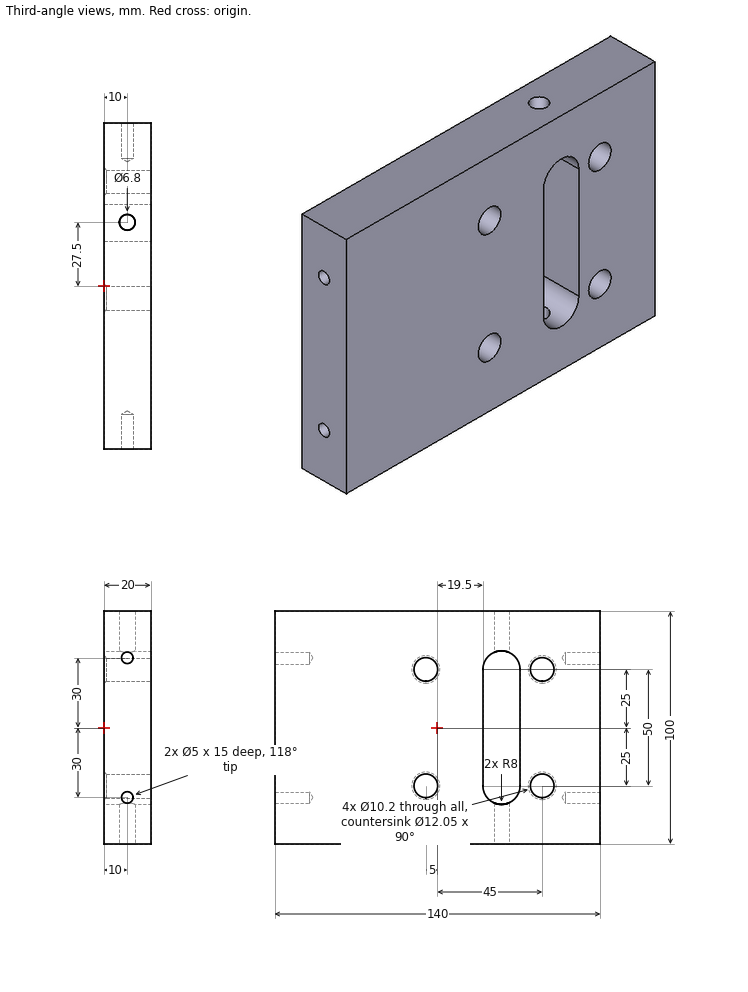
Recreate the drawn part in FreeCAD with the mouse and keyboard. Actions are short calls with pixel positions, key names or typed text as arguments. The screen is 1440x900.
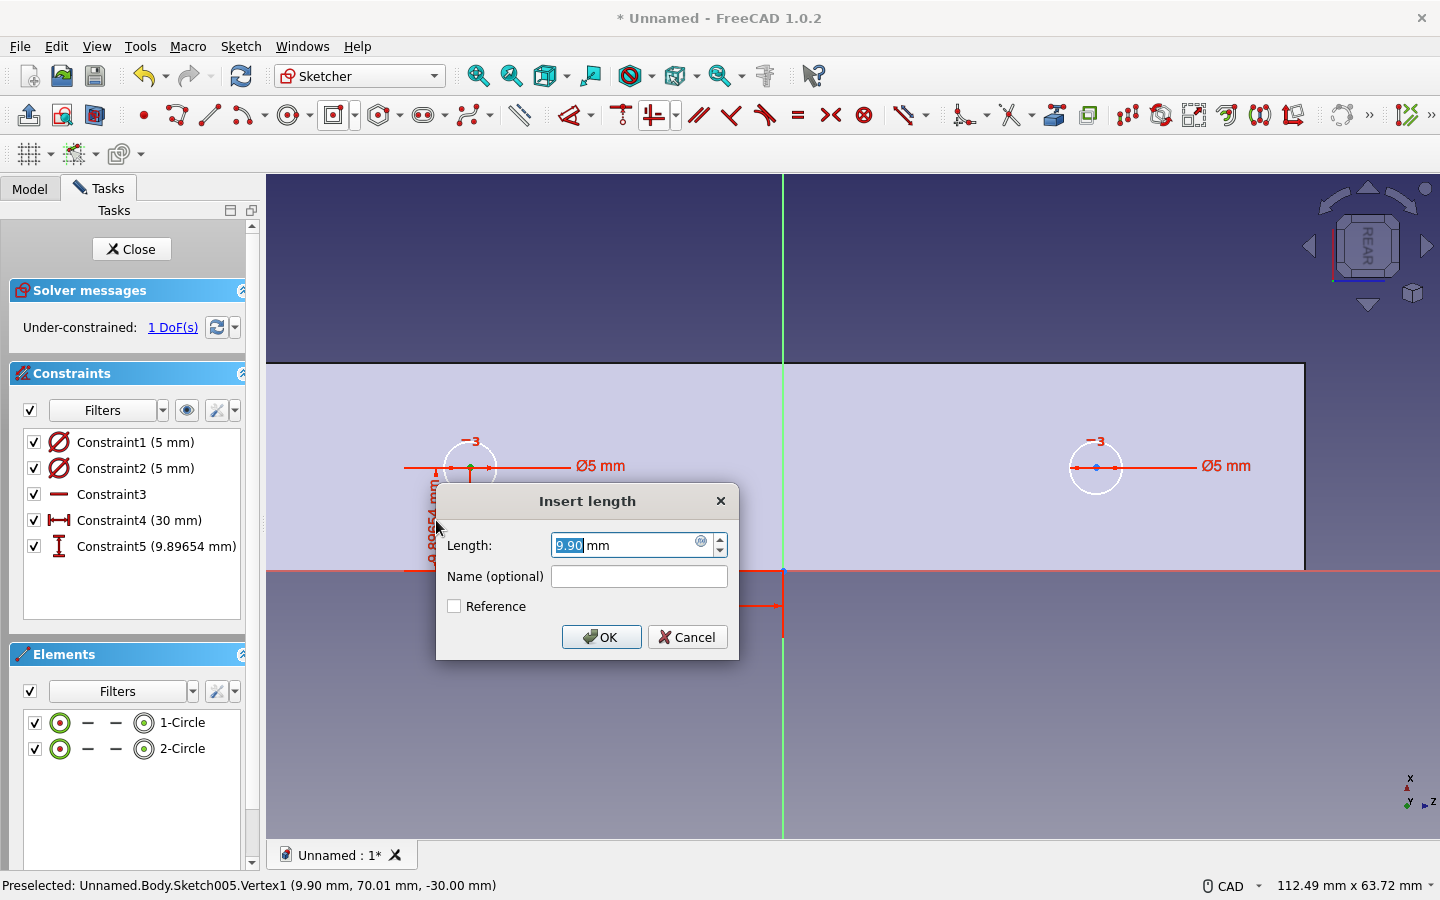
text(10)
key(Return)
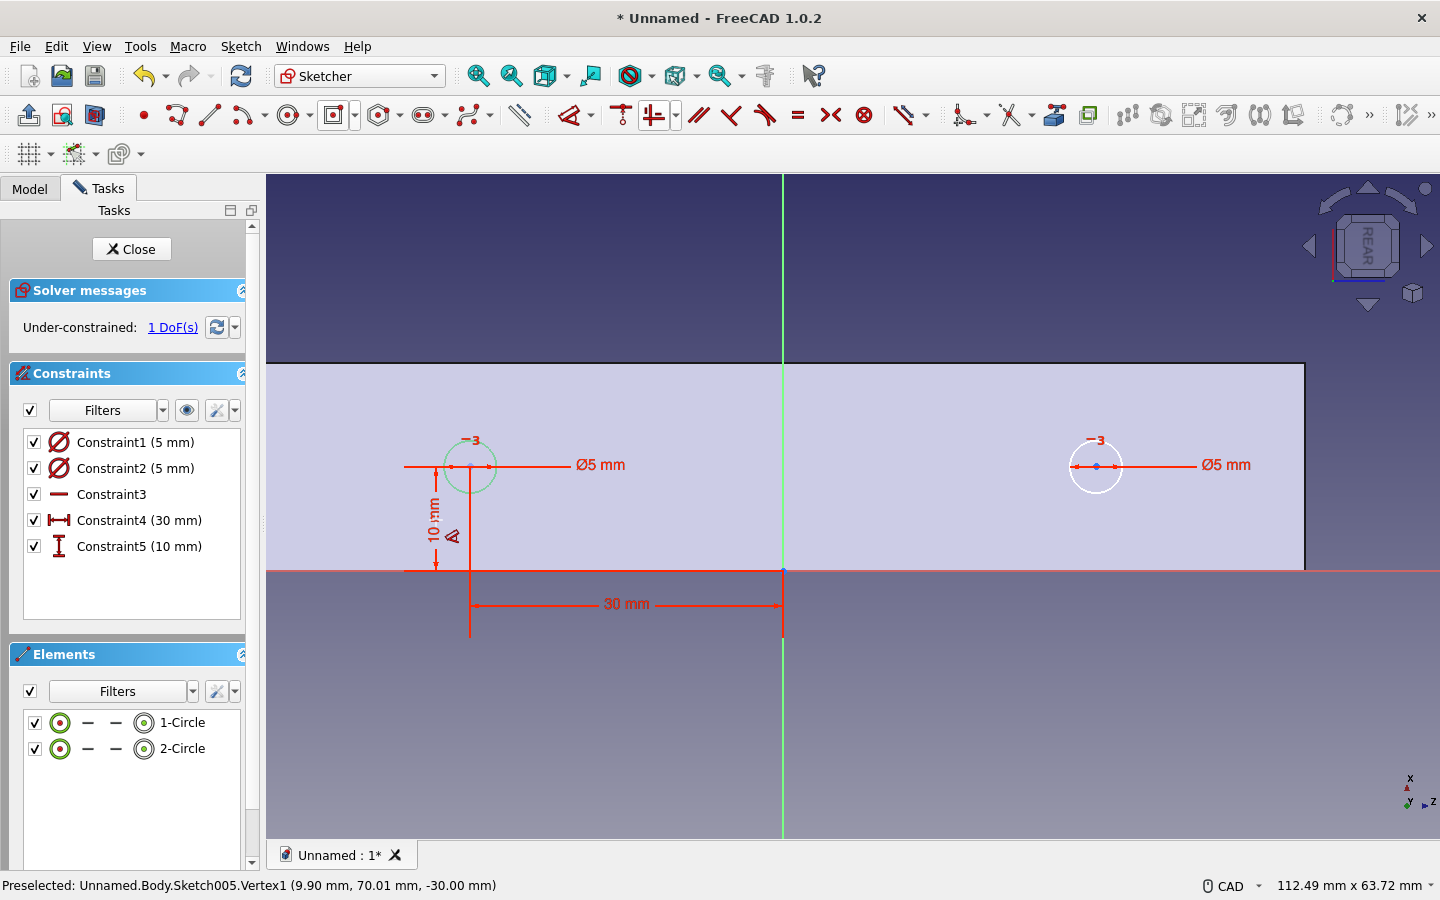
click(1096, 467)
click(940, 605)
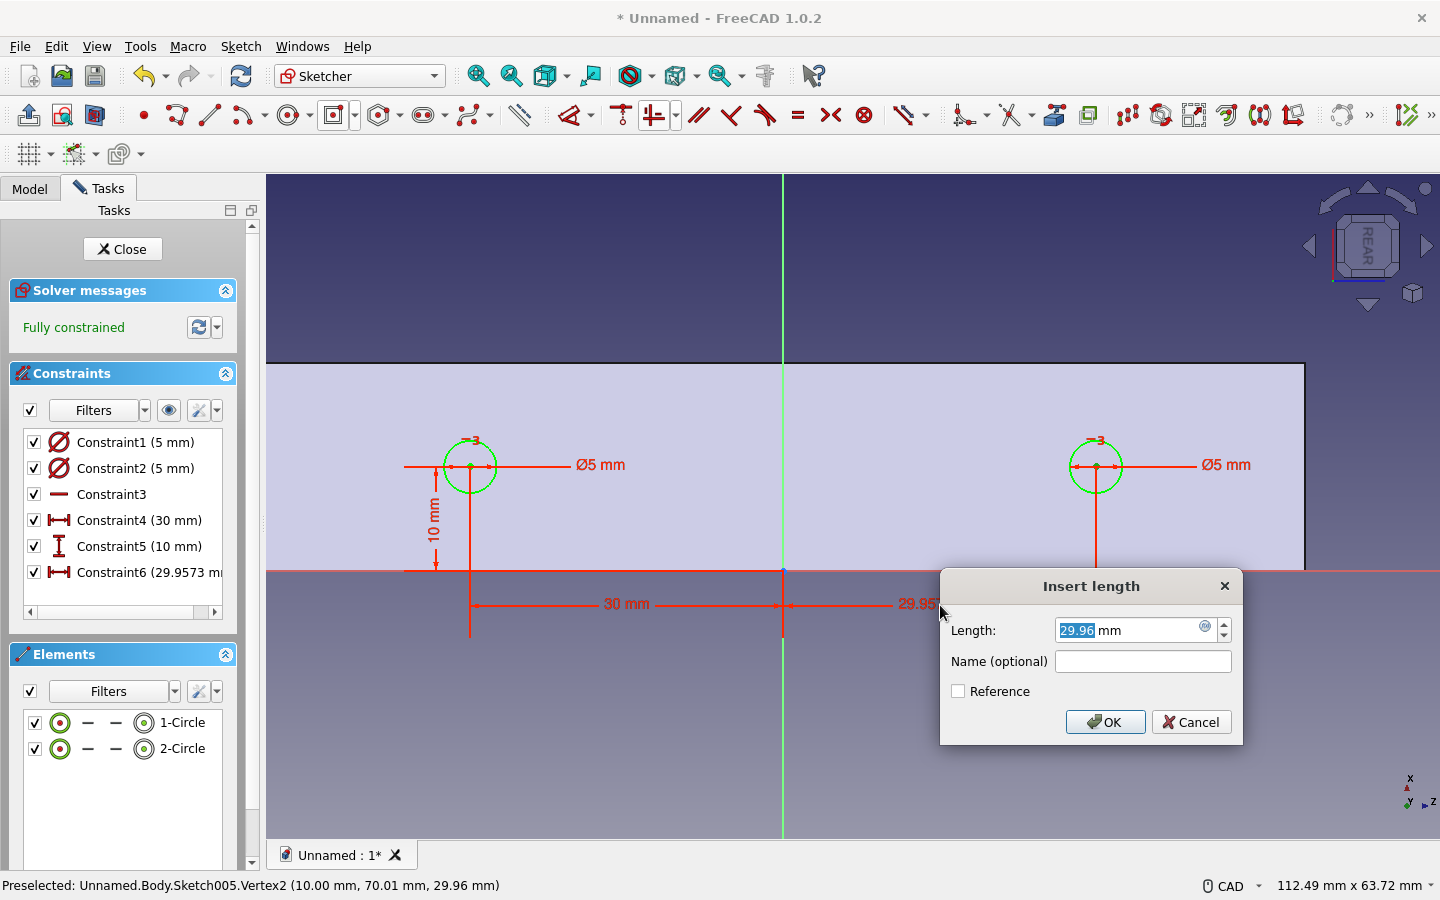
text(30)
key(Return)
key(Escape)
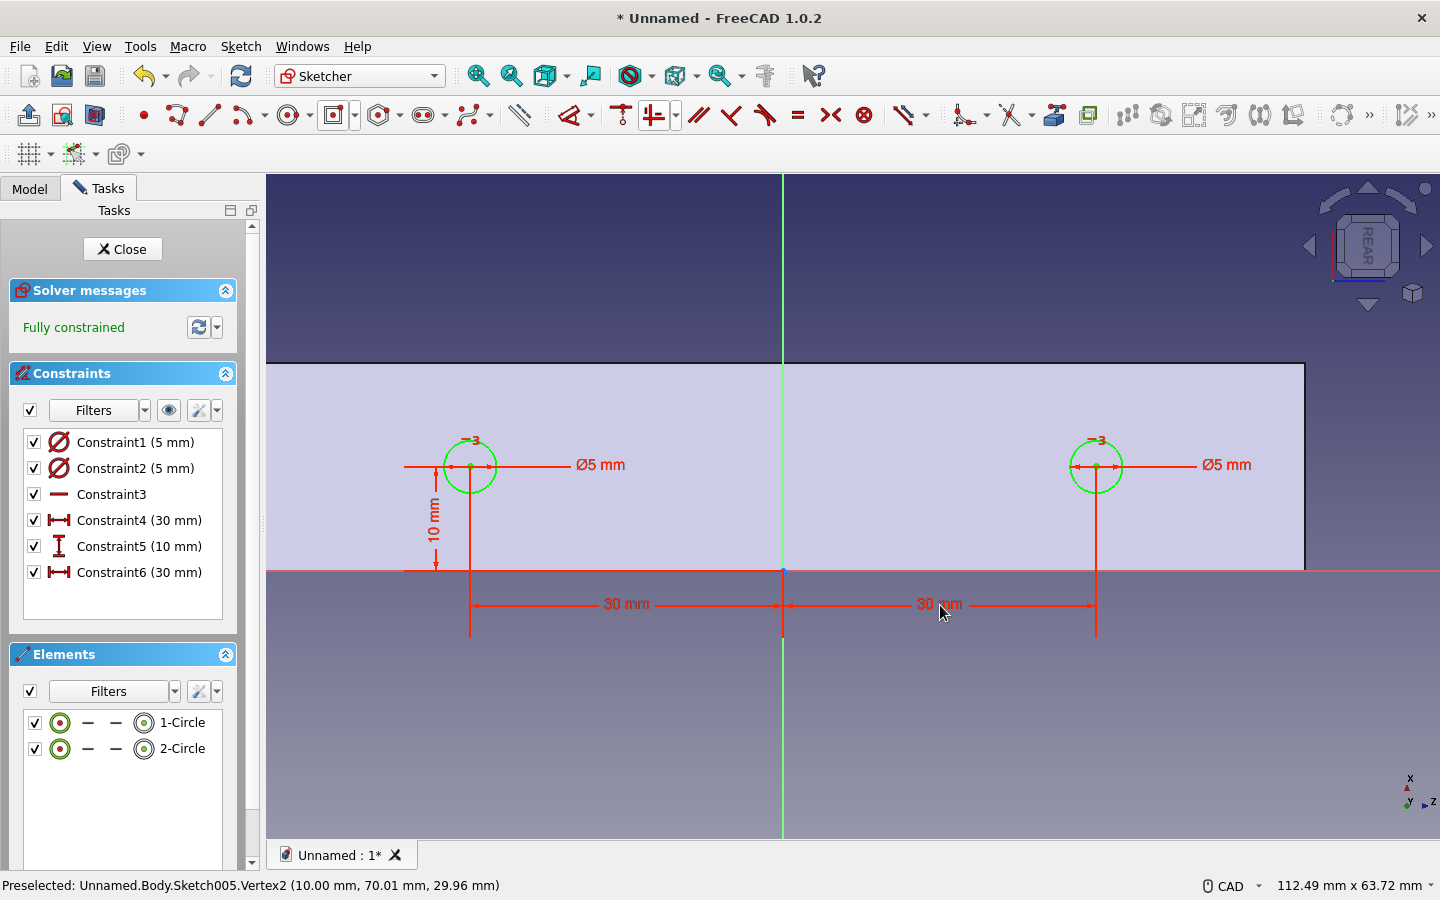
click(123, 249)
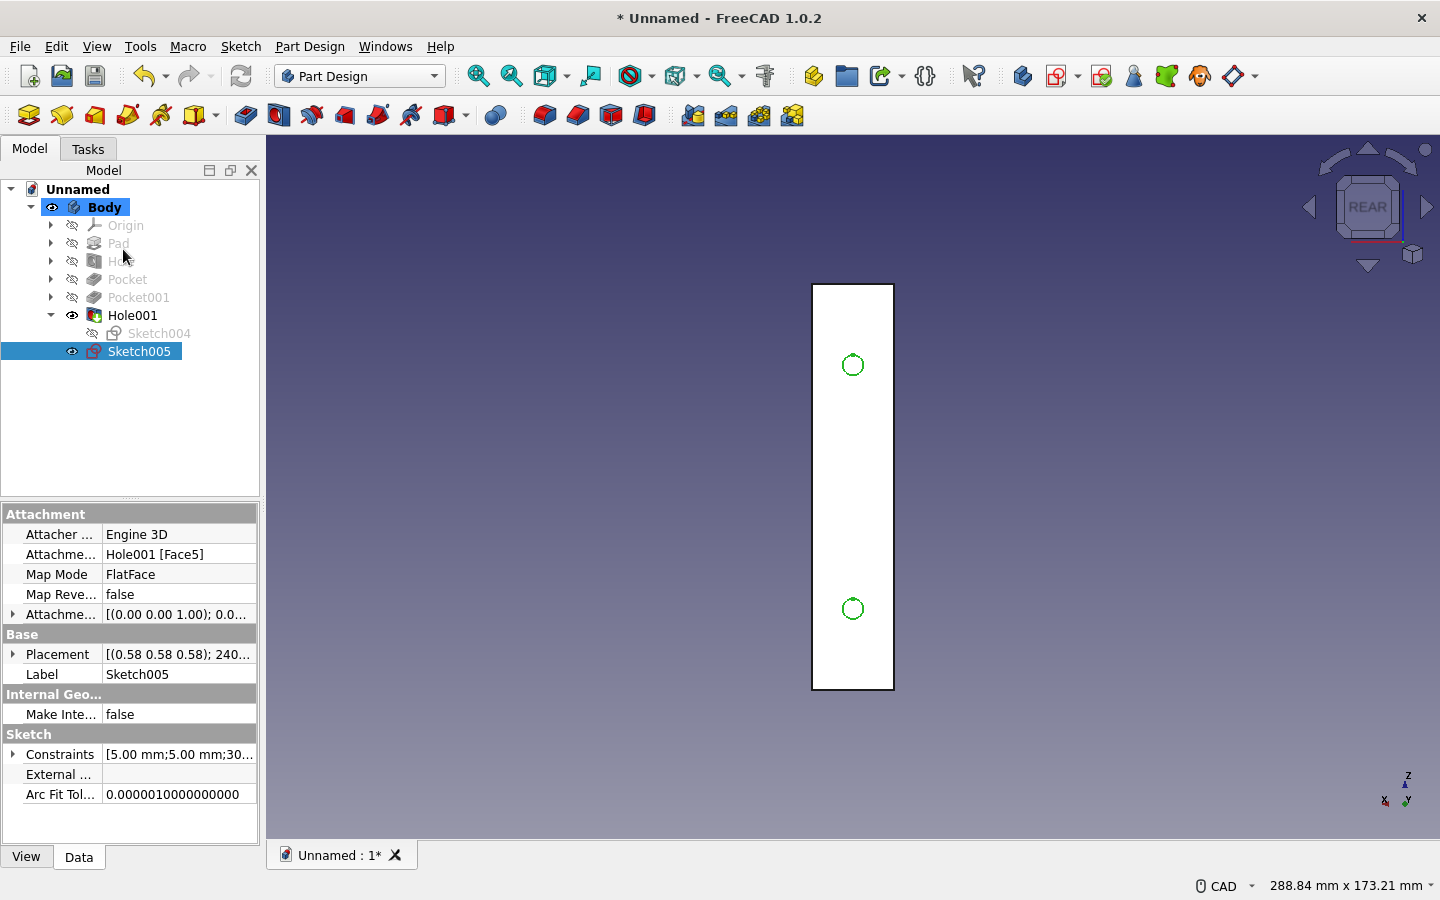
click(279, 116)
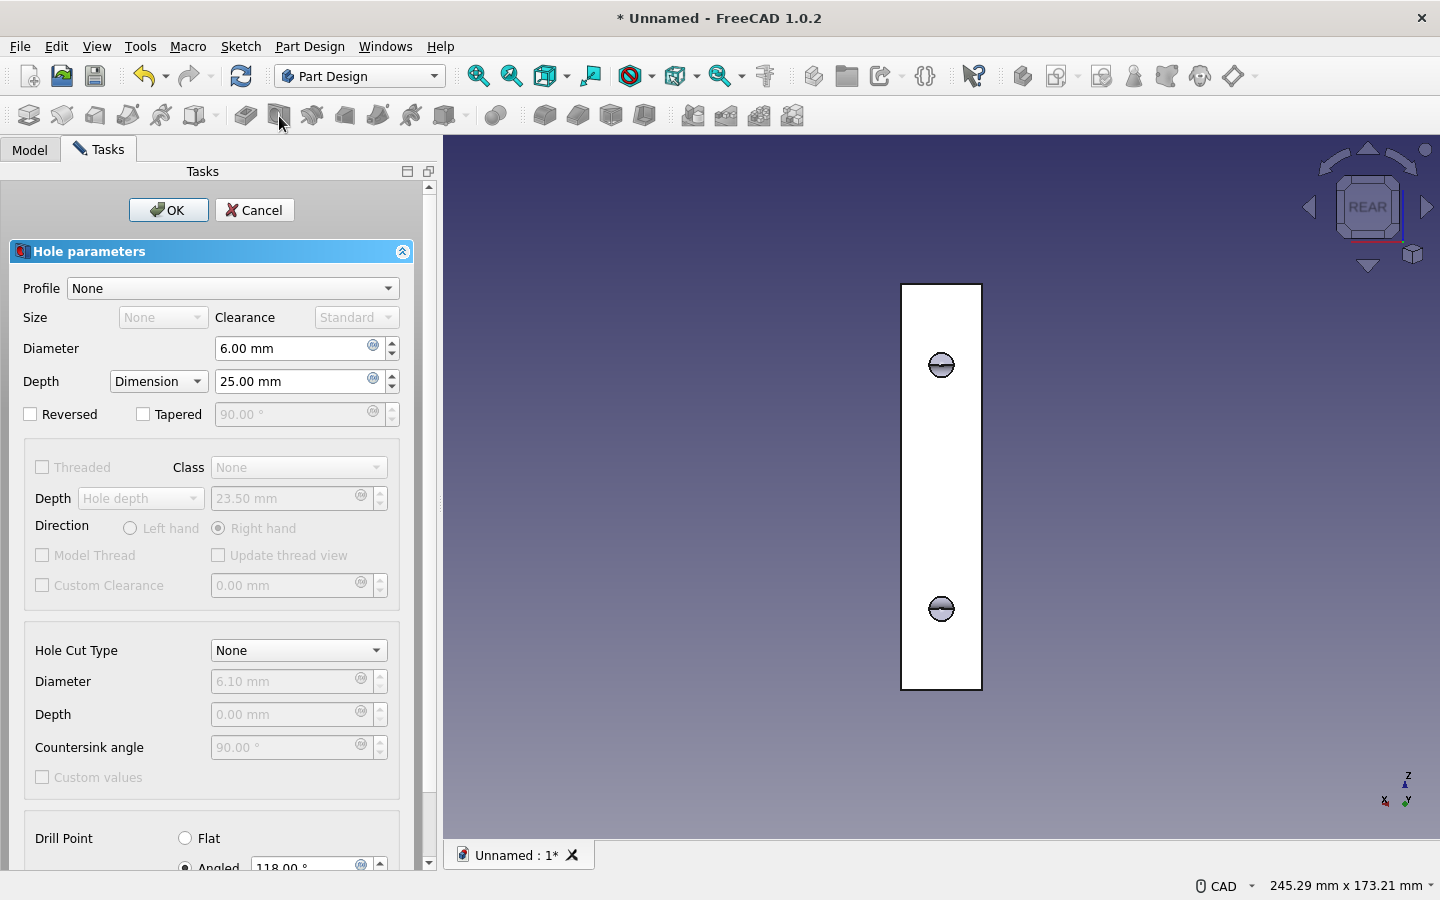
triple_click(300, 348)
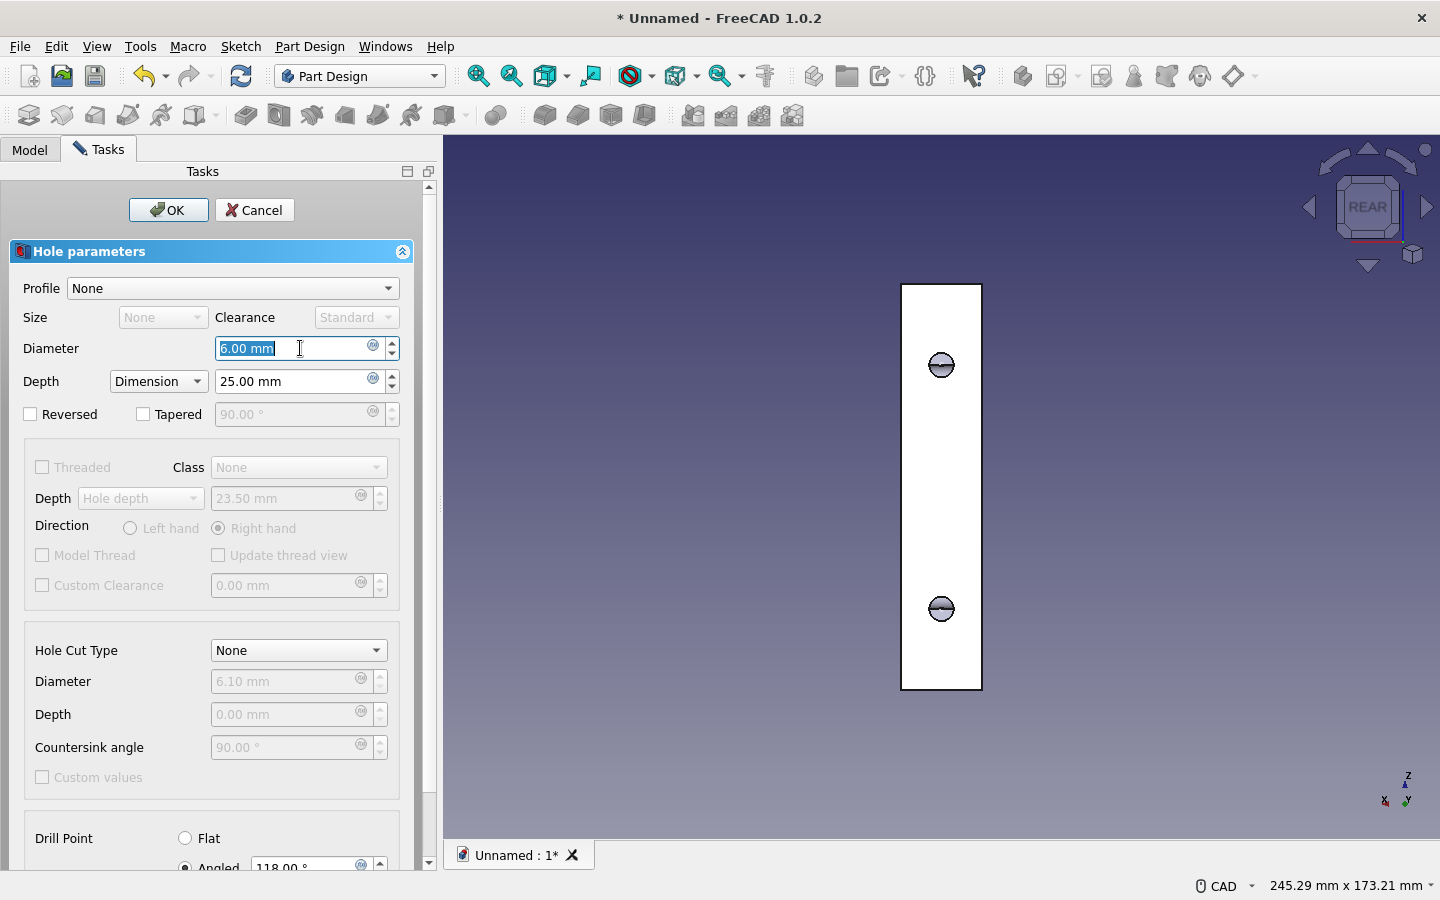
text(5)
key(Tab)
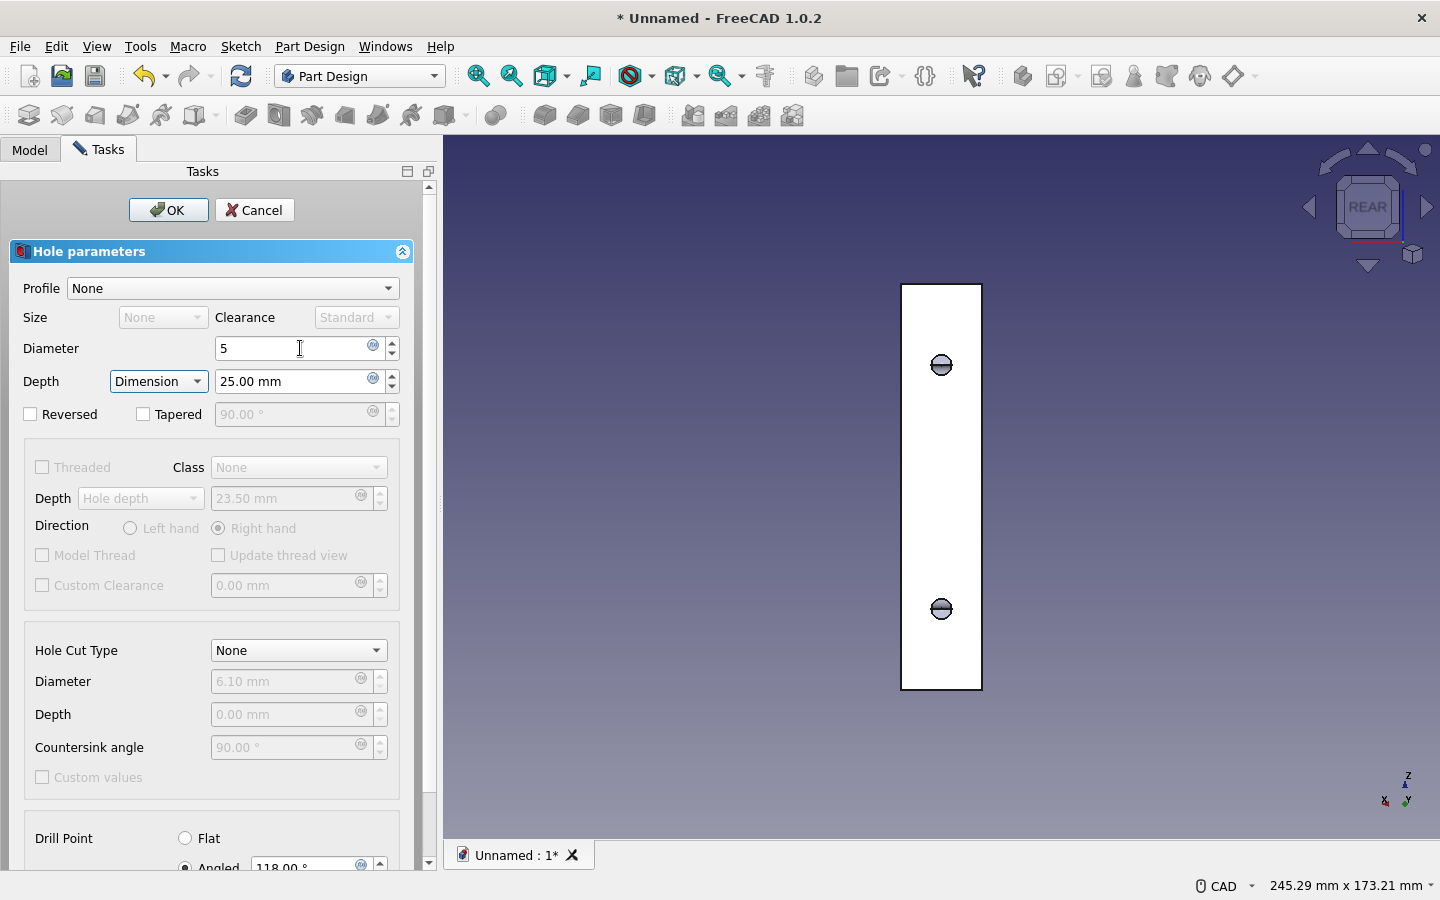
triple_click(300, 382)